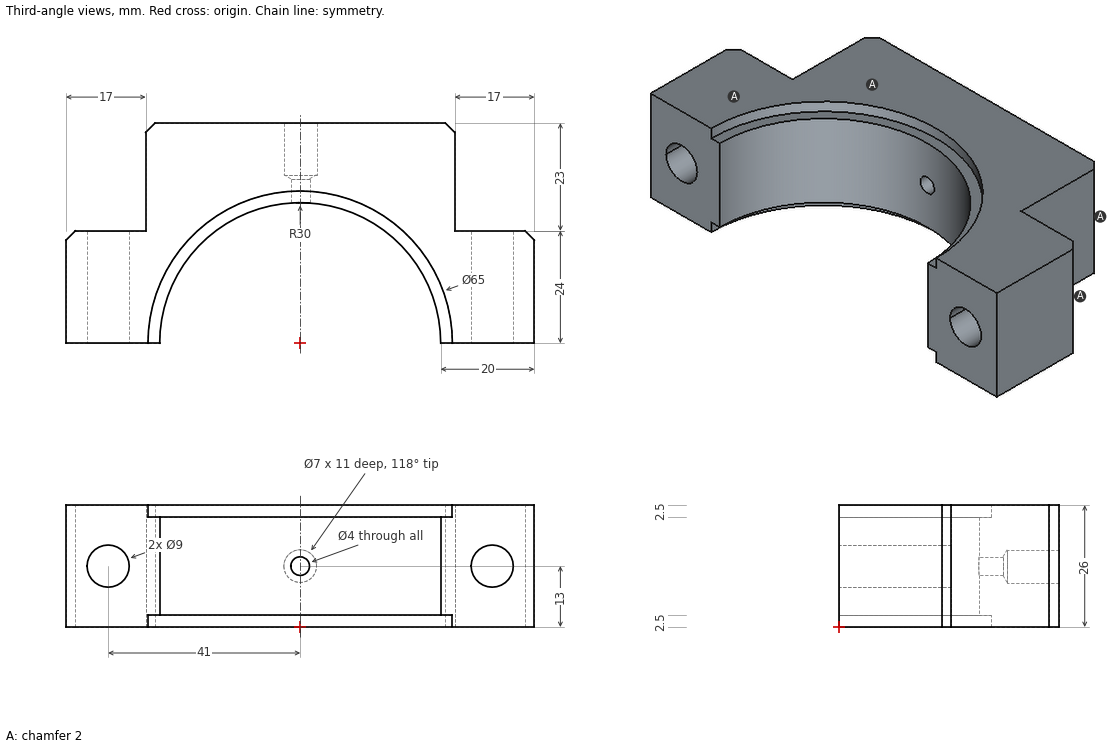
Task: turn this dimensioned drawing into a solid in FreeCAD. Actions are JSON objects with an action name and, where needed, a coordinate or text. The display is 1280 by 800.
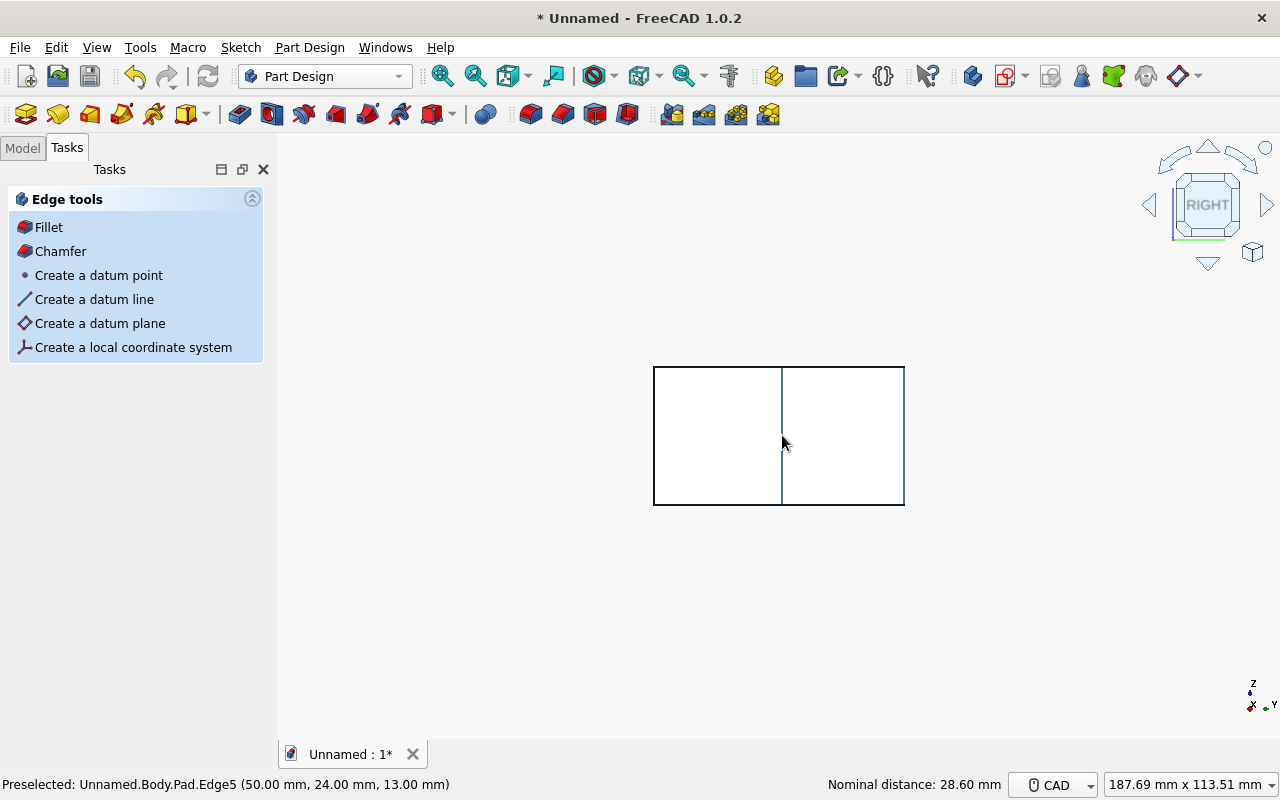
{"action": "key", "text": "5"}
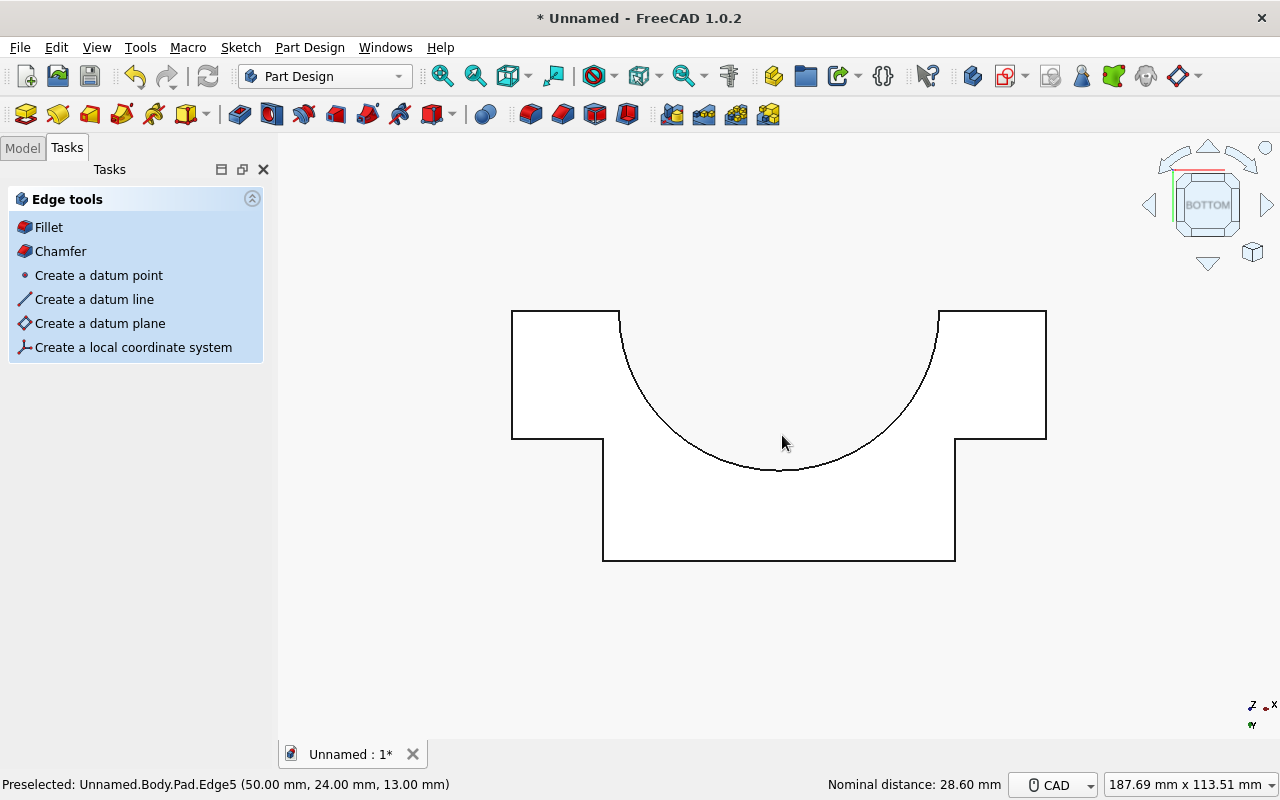
{"action": "key", "text": "4"}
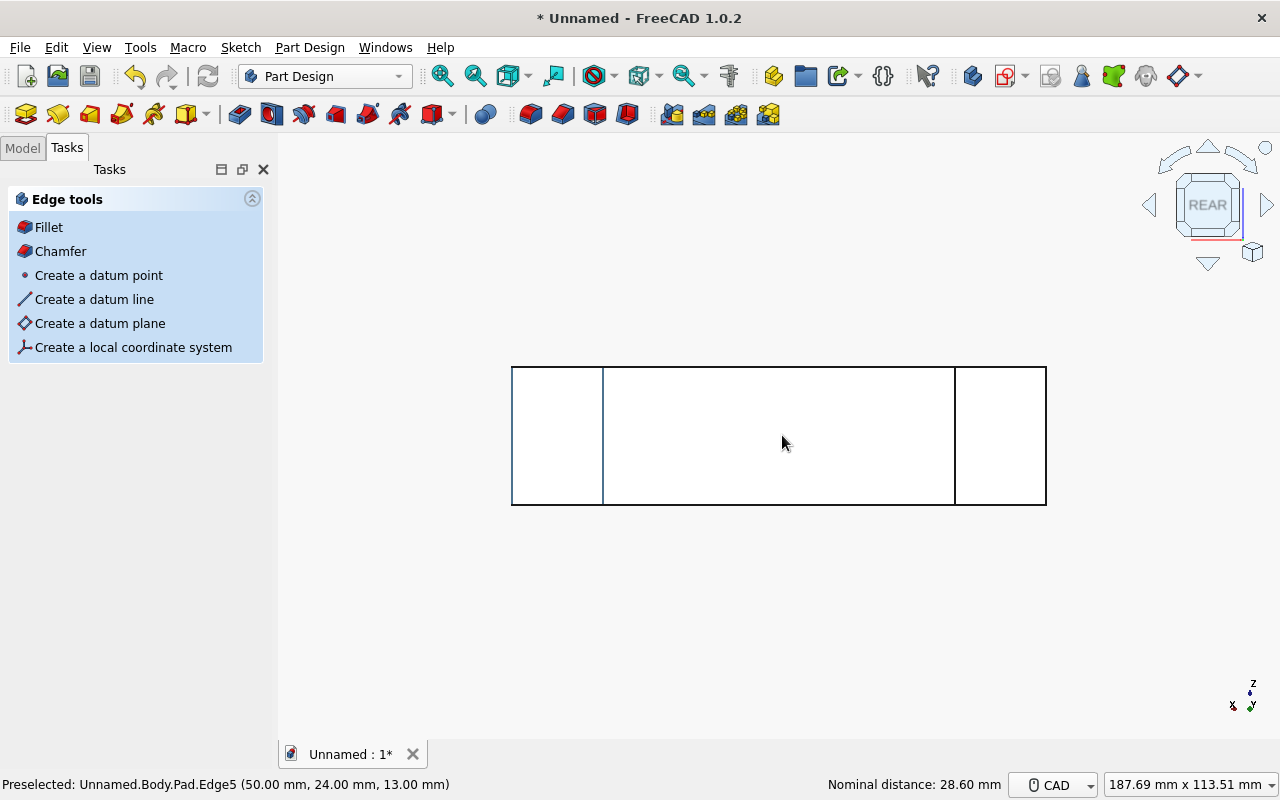
{"action": "left_click", "coordinate": [1046, 435], "text": "ctrl"}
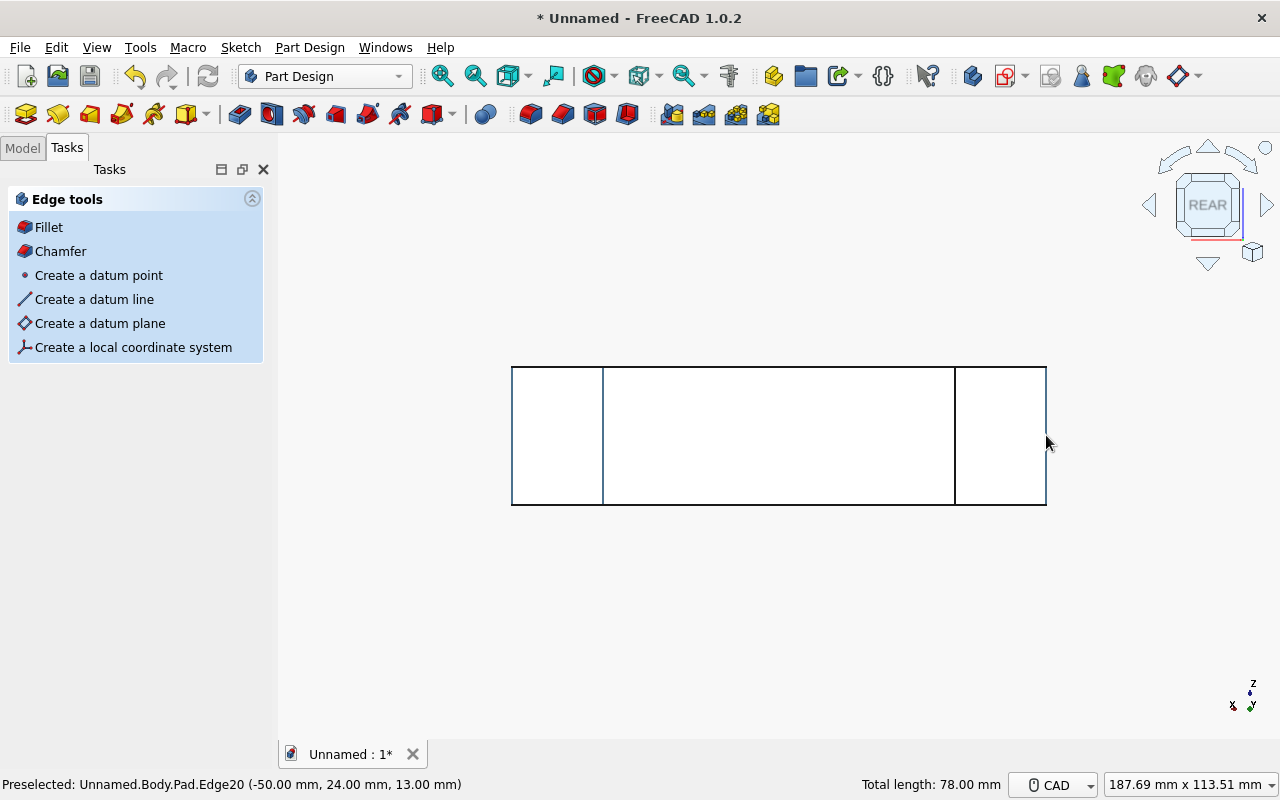
{"action": "left_click", "coordinate": [955, 435], "text": "ctrl"}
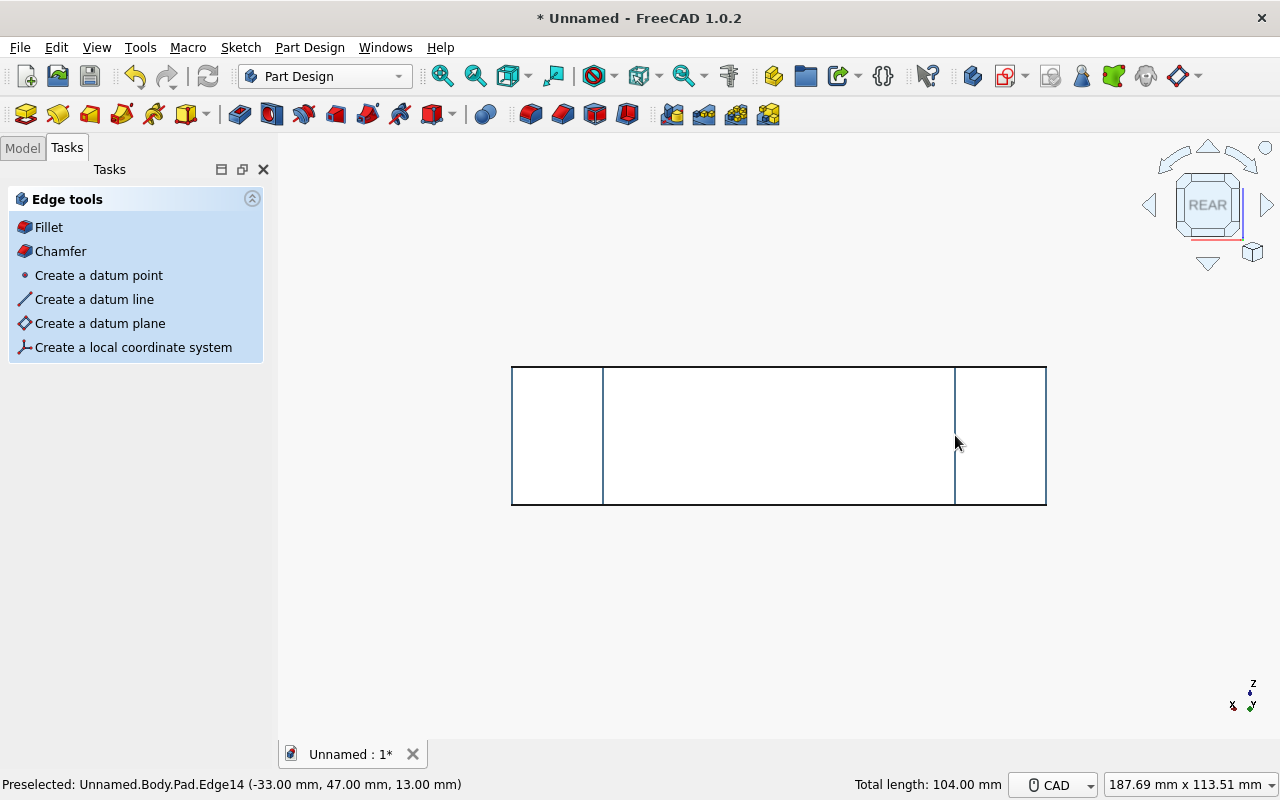
{"action": "left_click", "coordinate": [564, 114]}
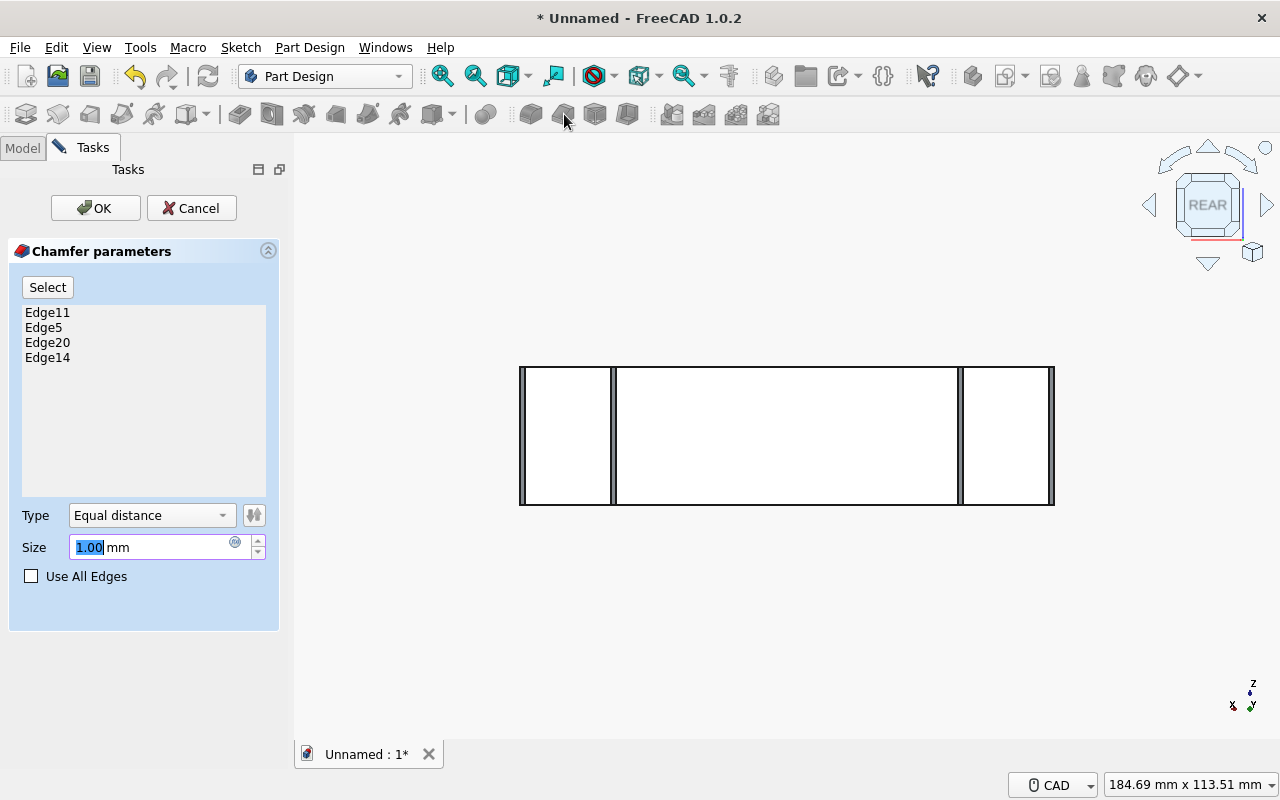
{"action": "type", "text": "2"}
{"action": "key", "text": "Tab"}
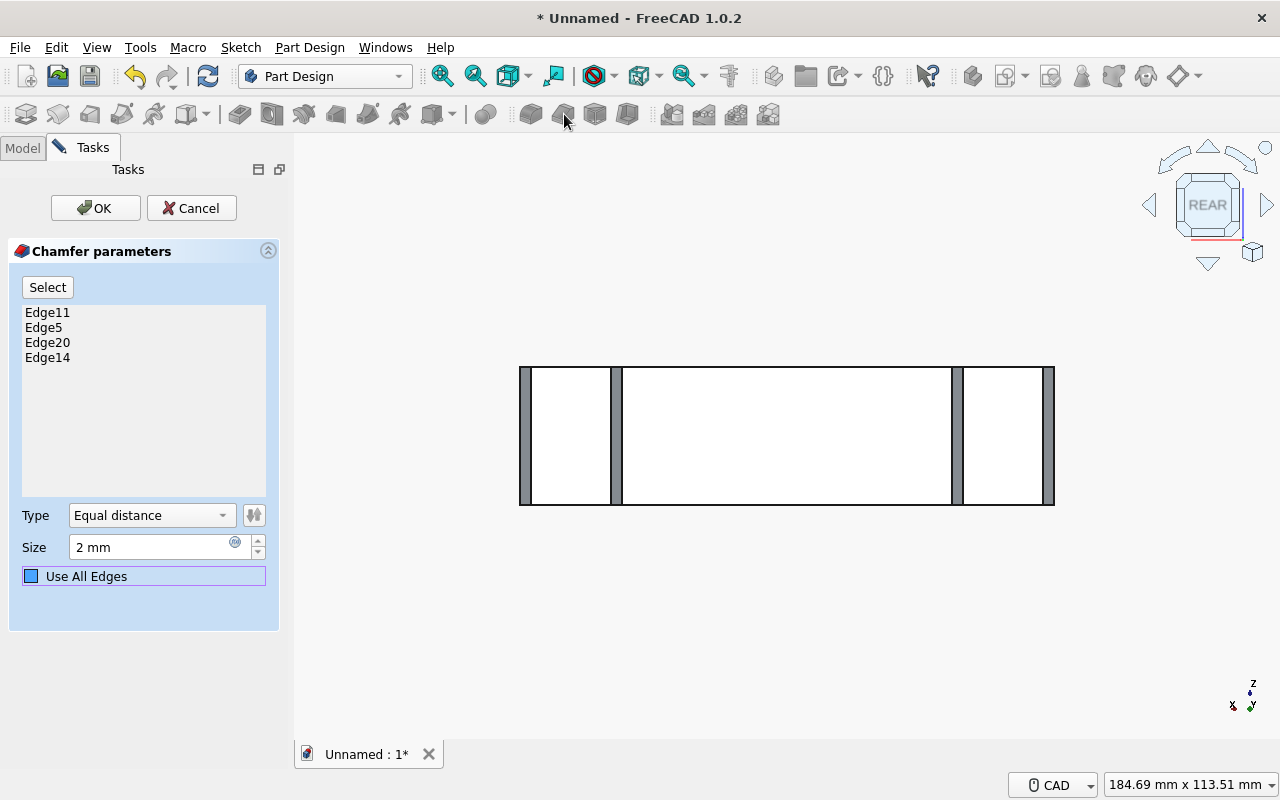
{"action": "left_click", "coordinate": [96, 208]}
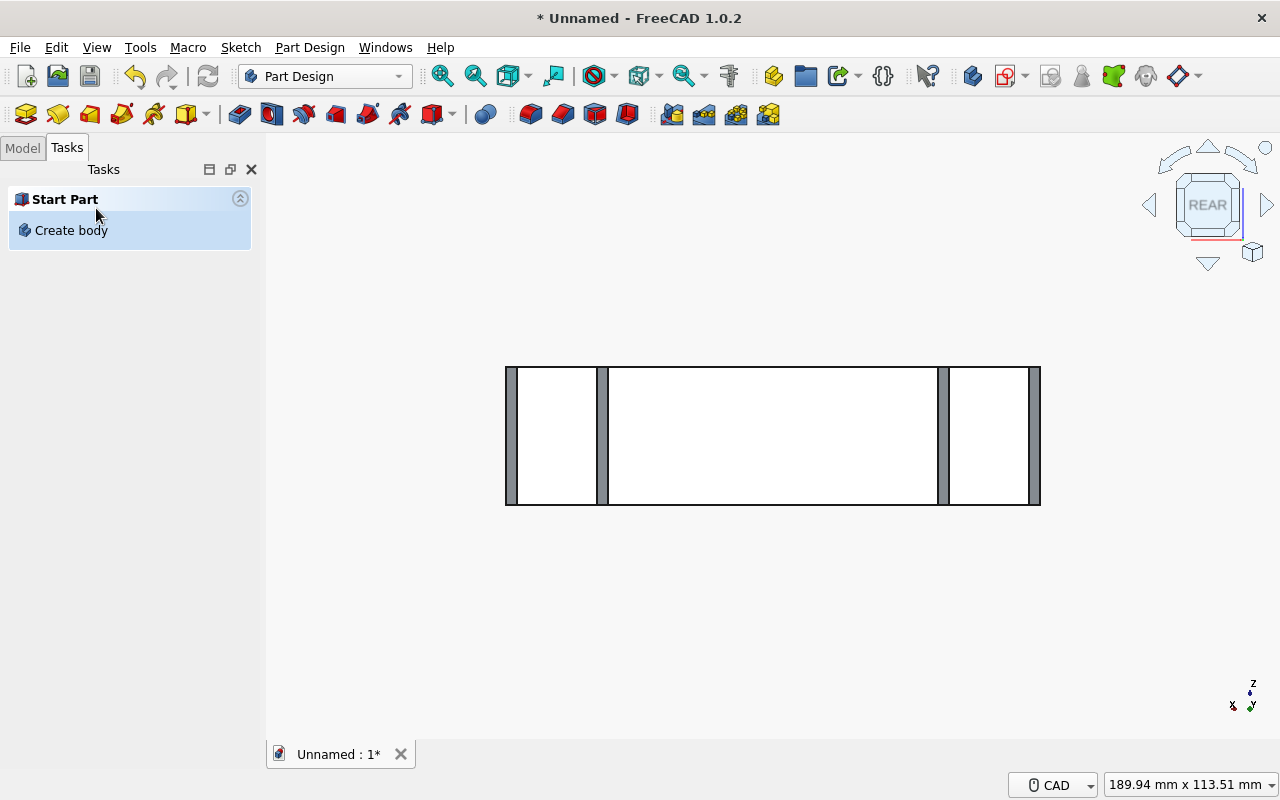
{"action": "left_click", "coordinate": [678, 435]}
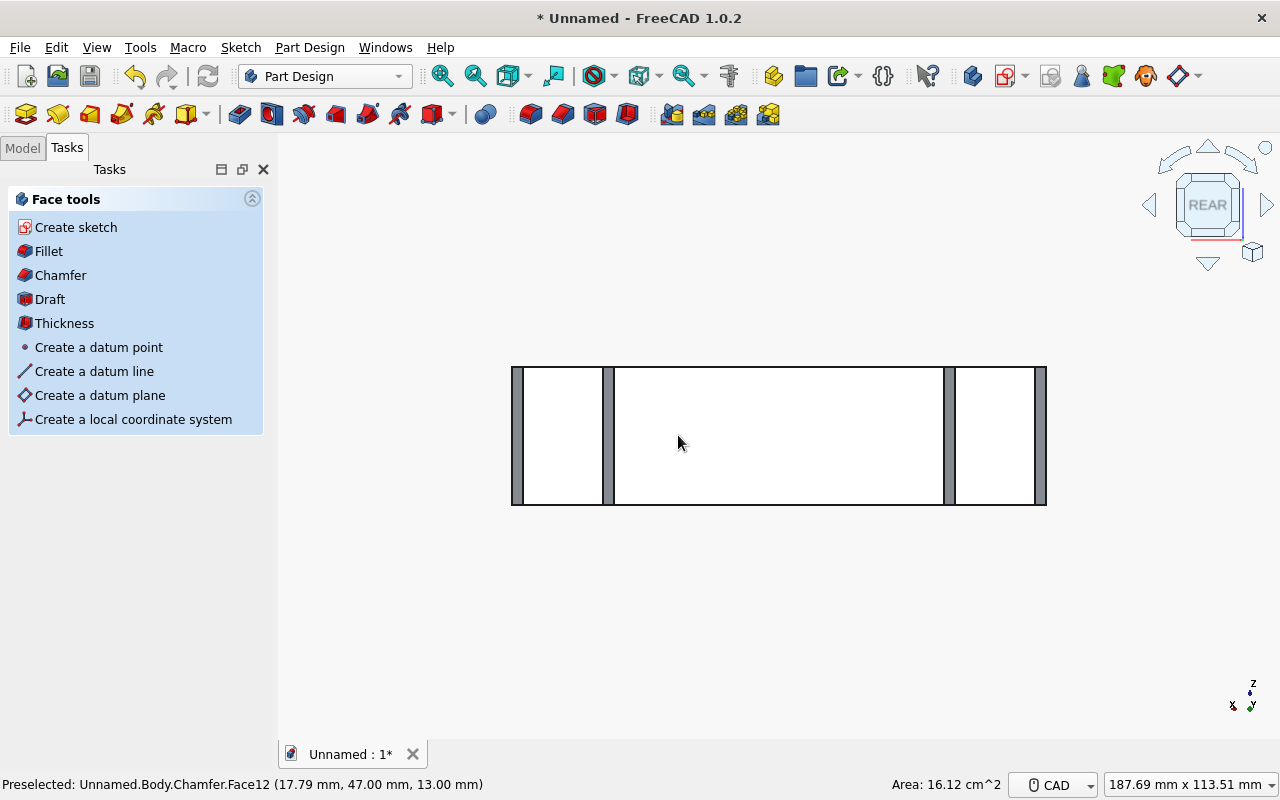
{"action": "left_click", "coordinate": [1006, 76]}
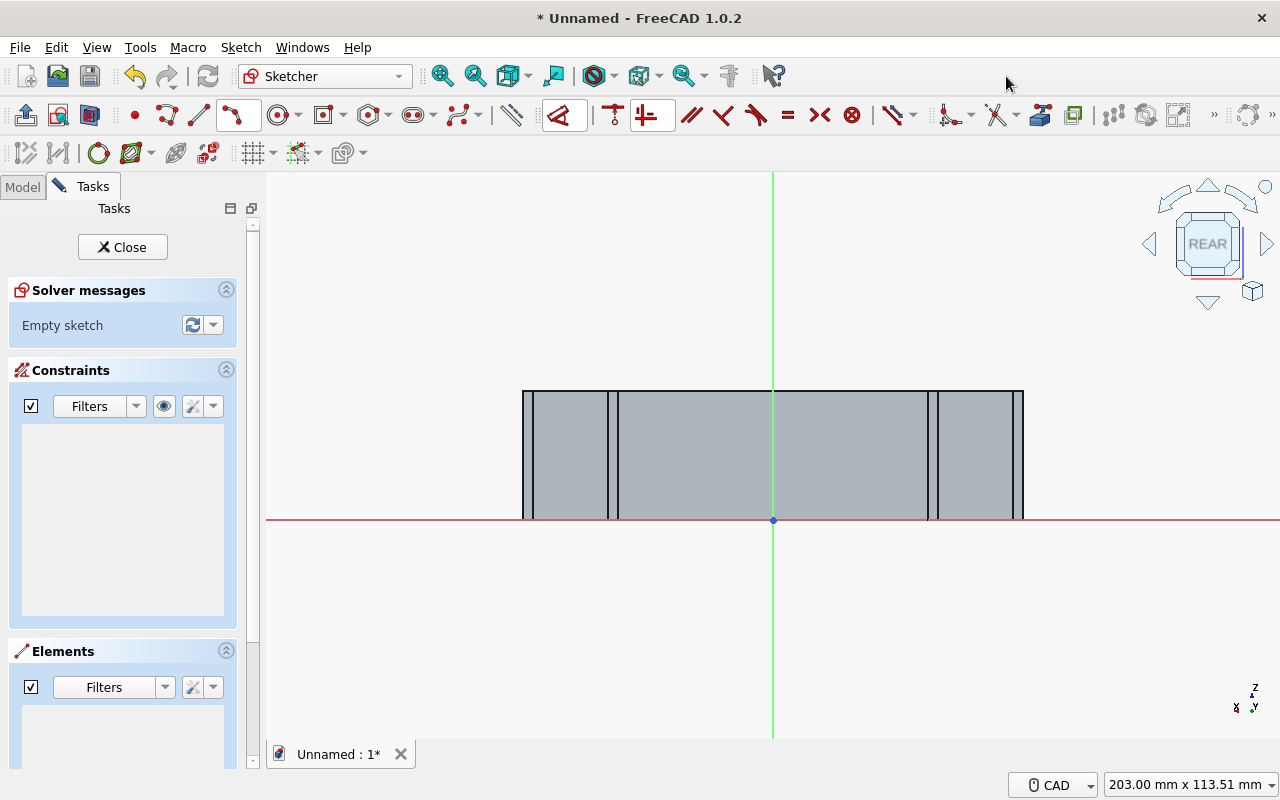
{"action": "scroll", "coordinate": [795, 487], "scroll_direction": "up", "scroll_amount": 7}